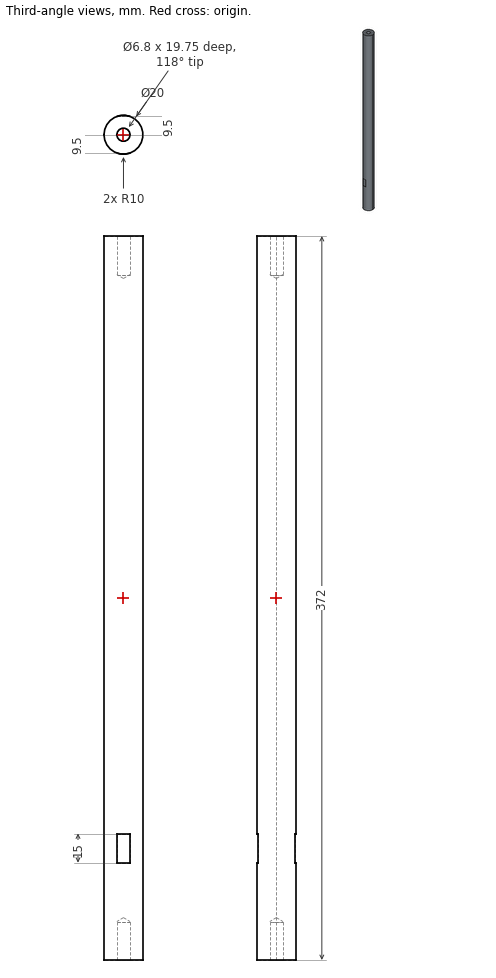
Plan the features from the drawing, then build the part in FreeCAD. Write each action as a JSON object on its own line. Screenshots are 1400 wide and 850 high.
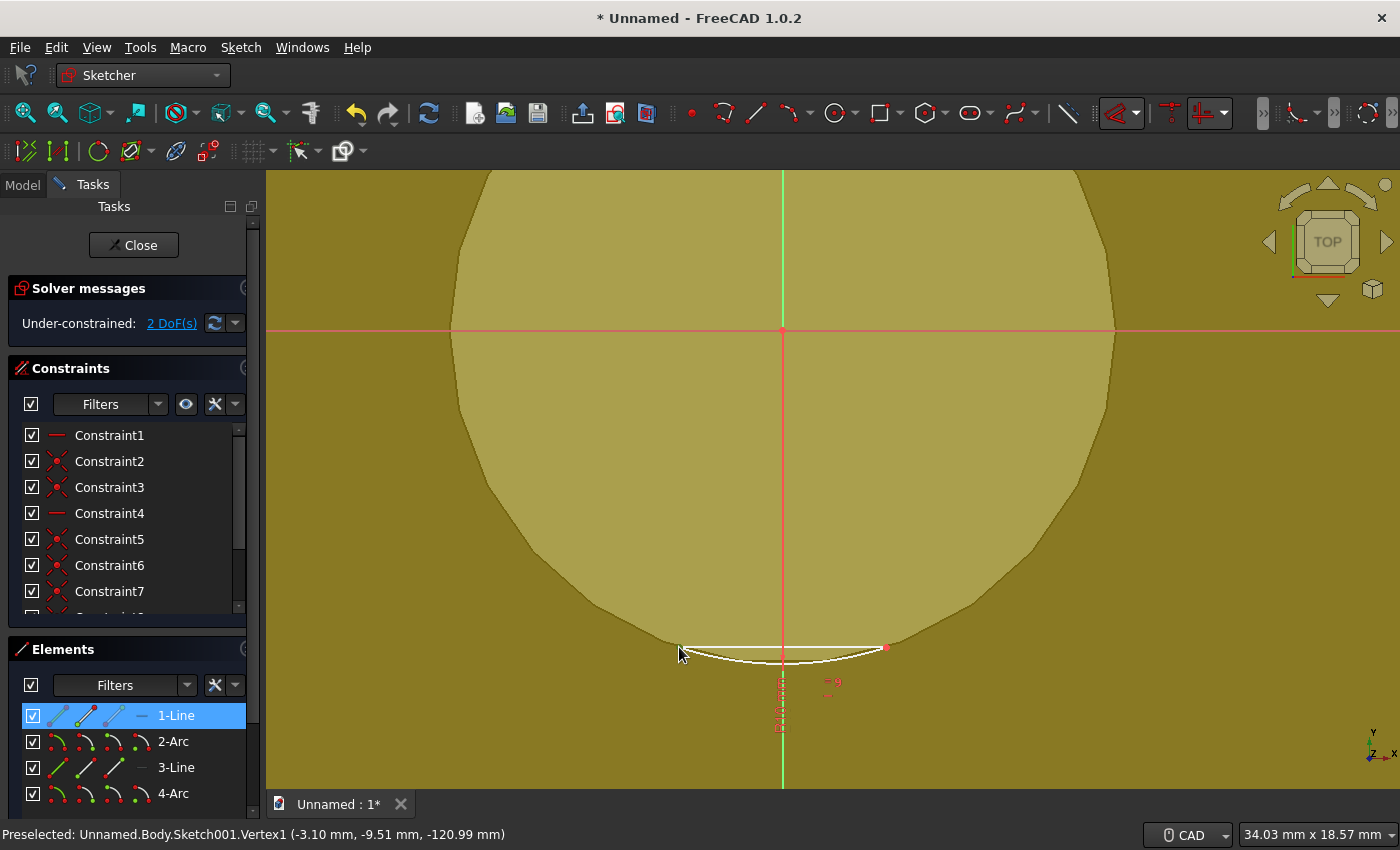
{"action": "key", "text": "i"}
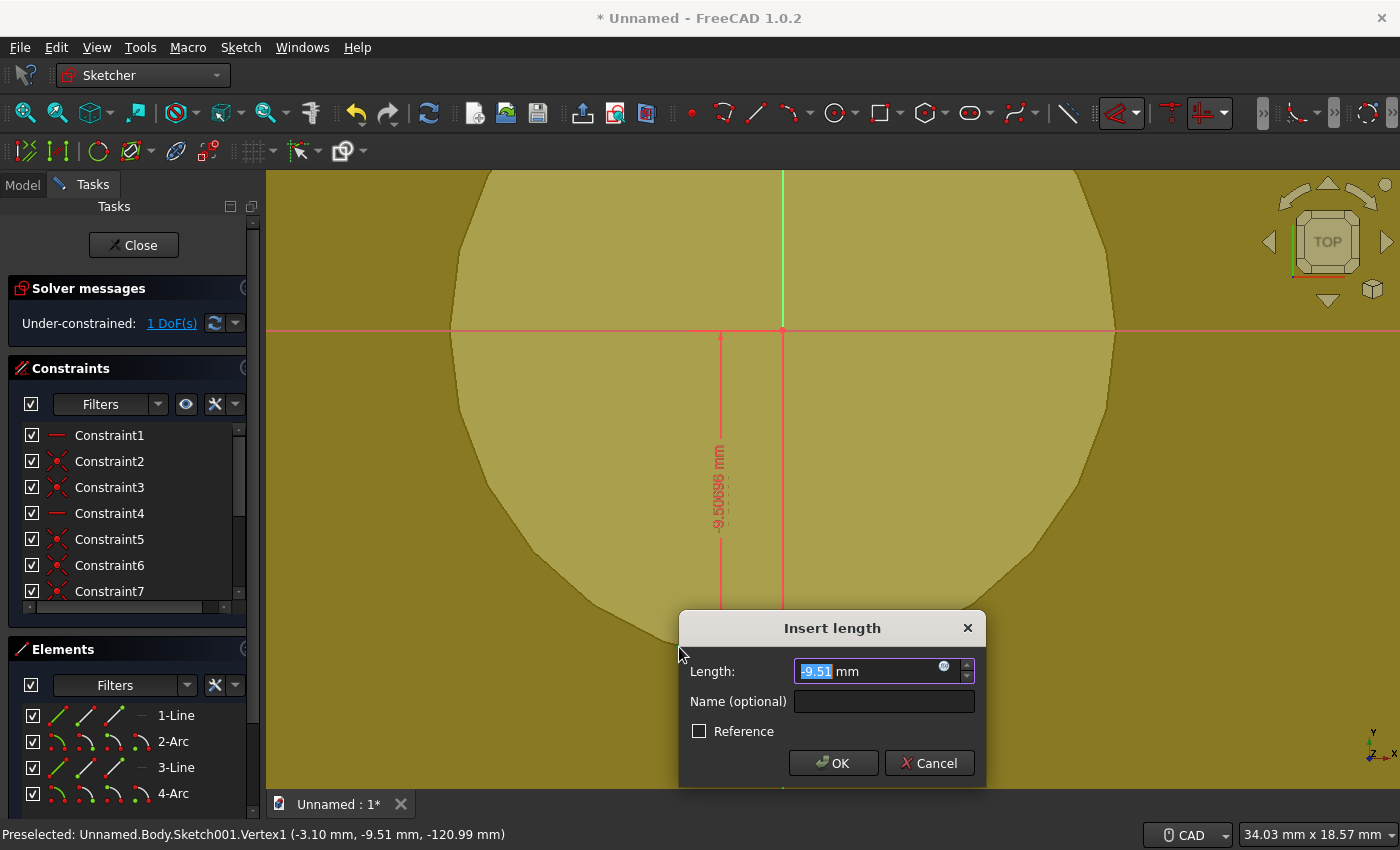
{"action": "type", "text": "-9.5"}
{"action": "key", "text": "Return"}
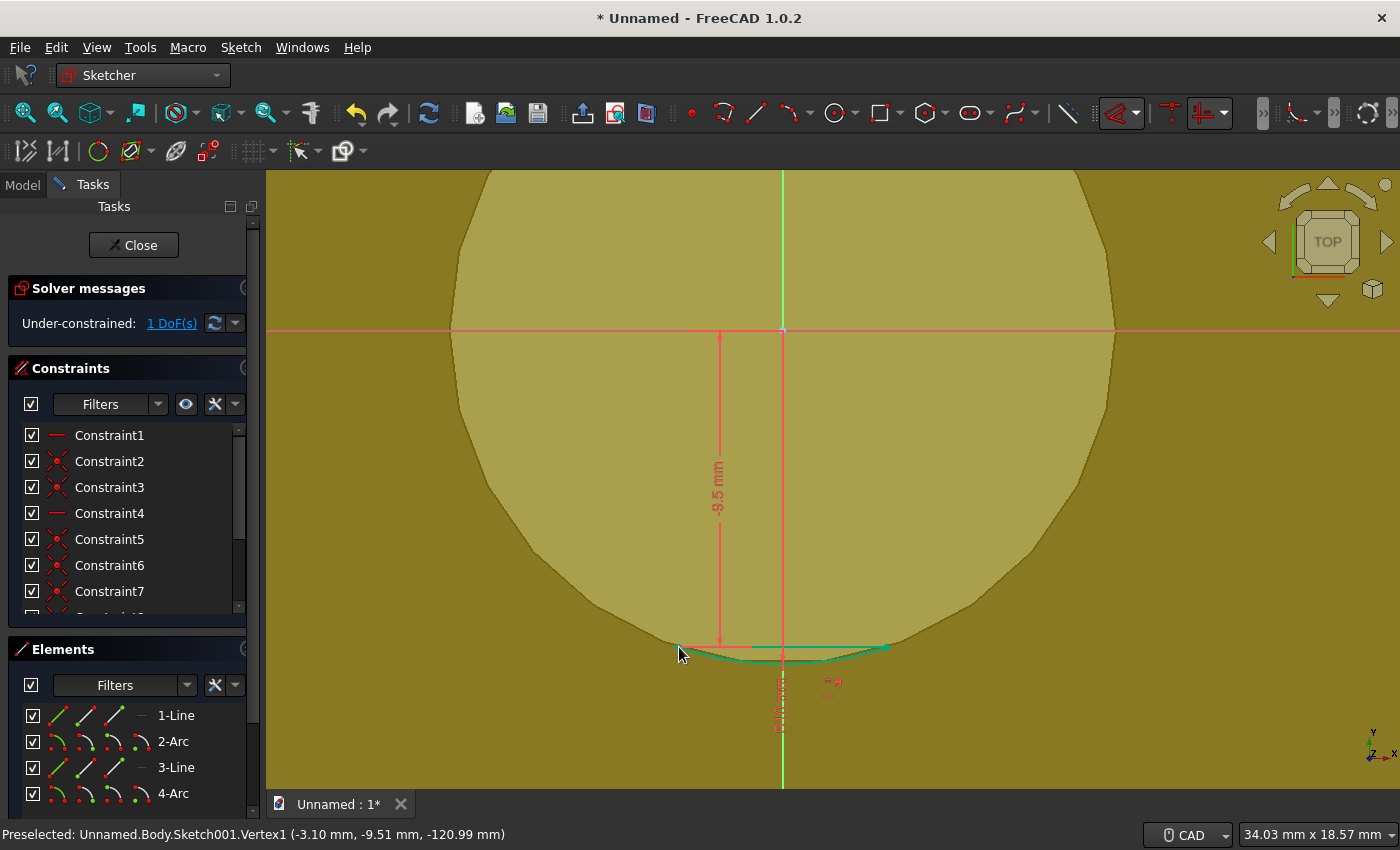
{"action": "scroll", "coordinate": [742, 661], "scroll_direction": "down", "scroll_amount": 3}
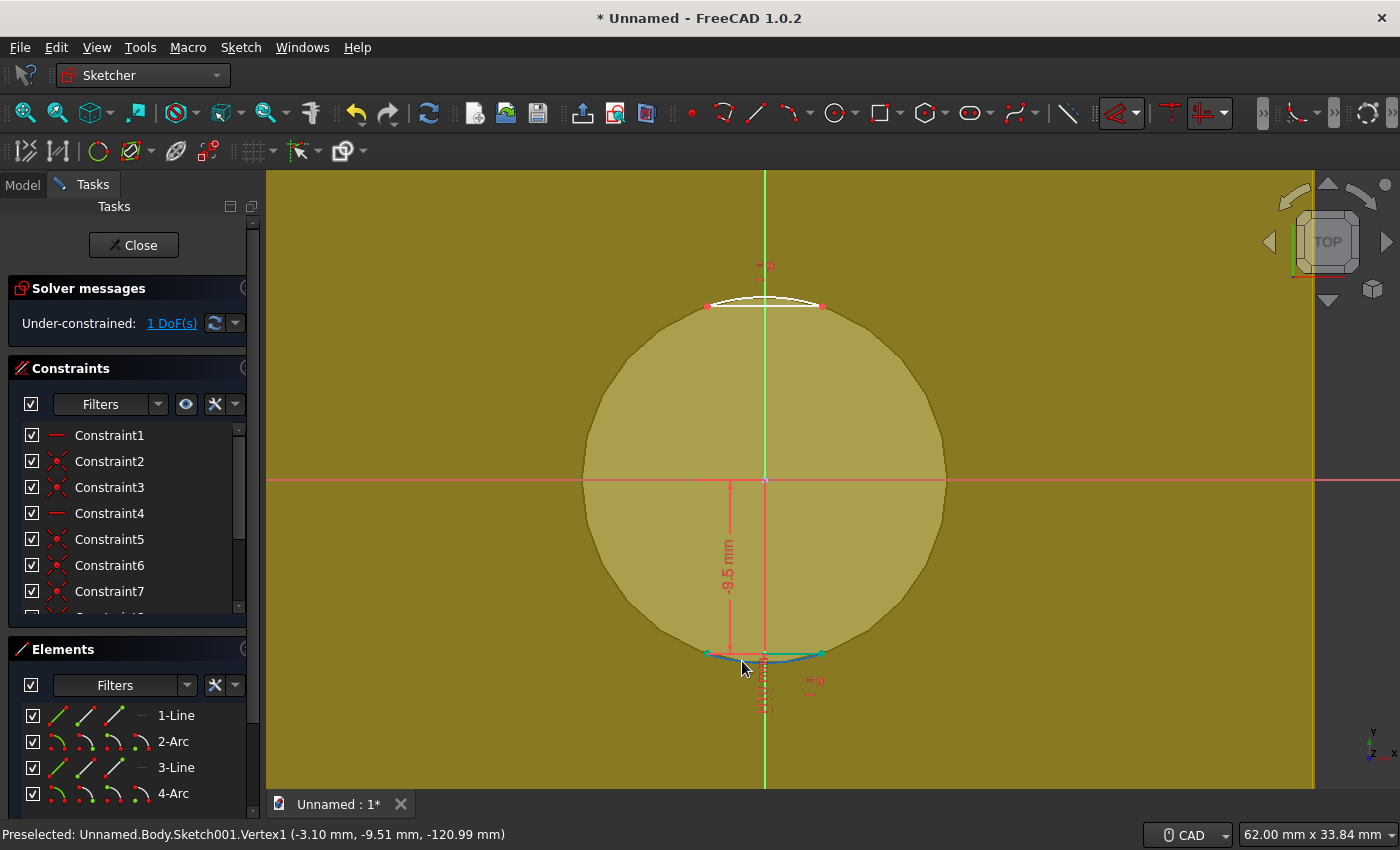
{"action": "left_click", "coordinate": [822, 306]}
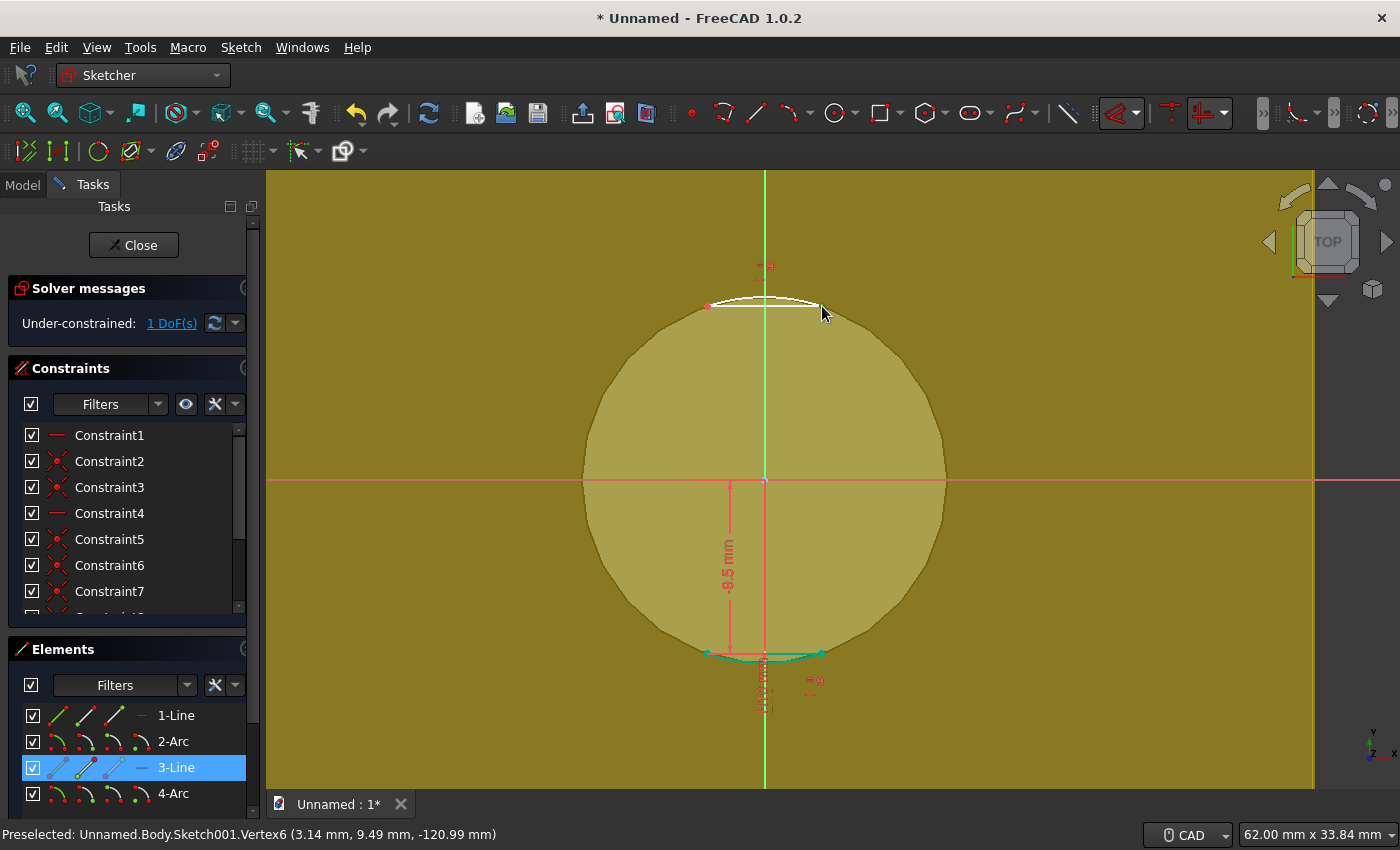
{"action": "left_click", "coordinate": [1138, 114]}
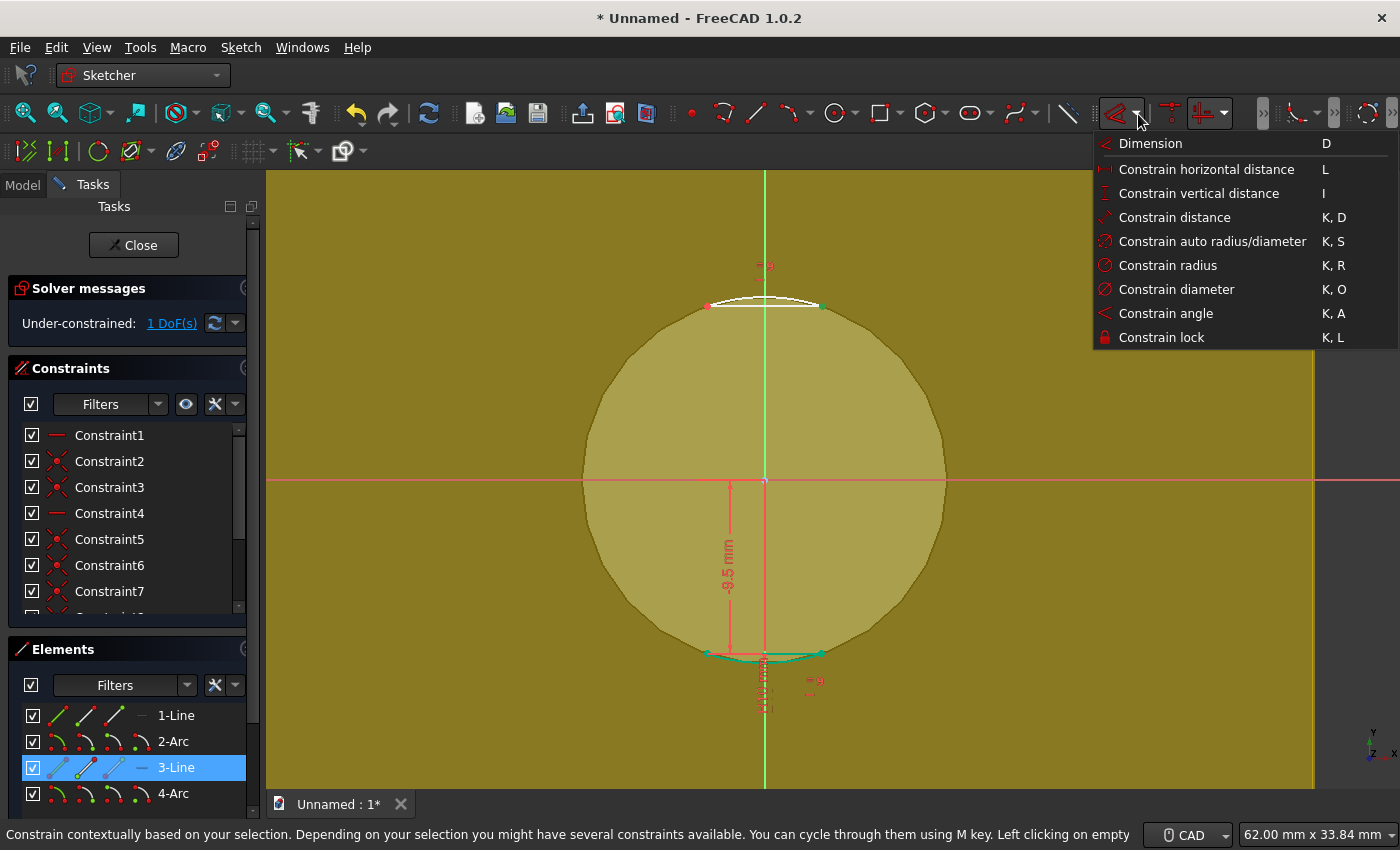
{"action": "left_click", "coordinate": [1246, 193]}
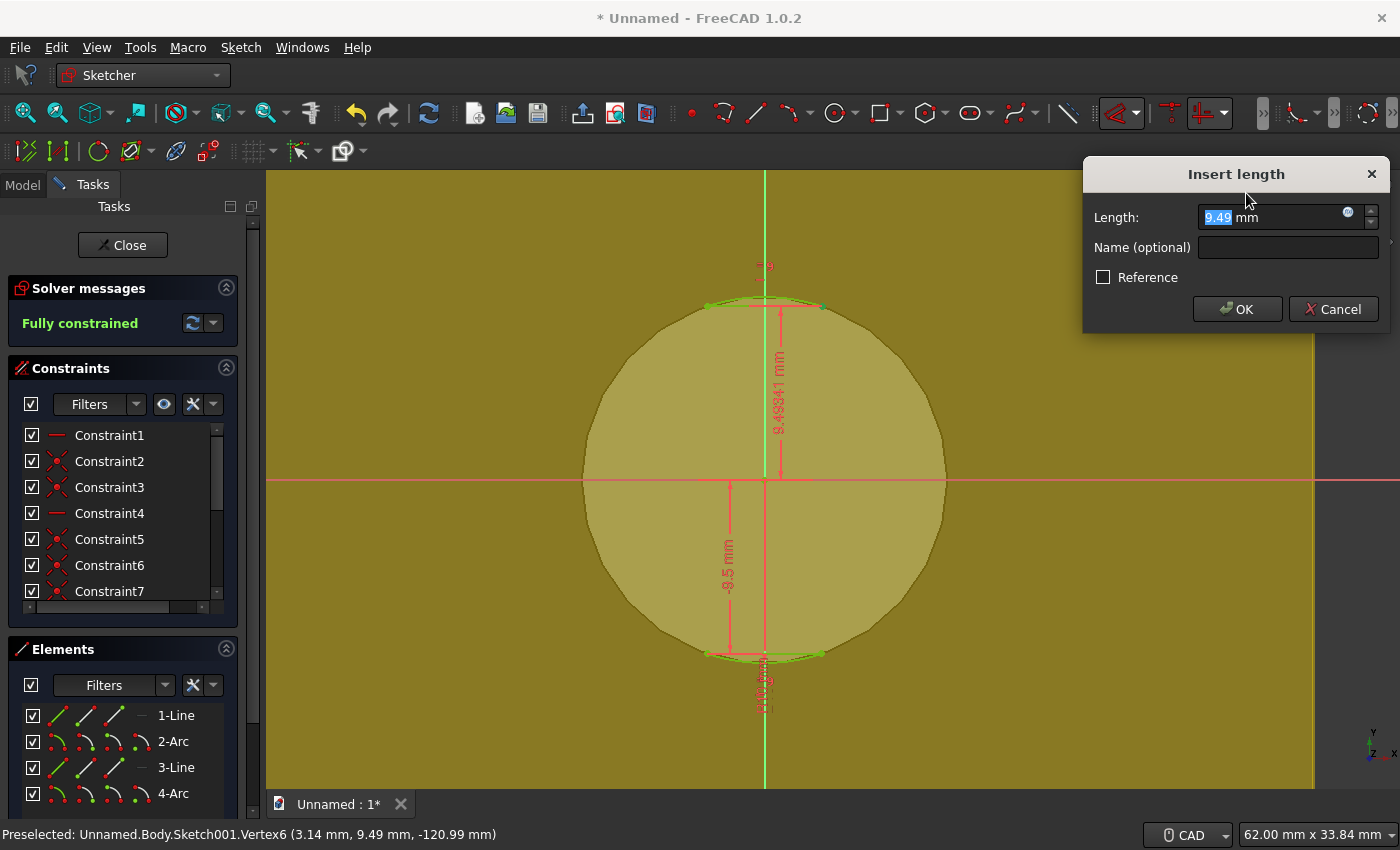
{"action": "type", "text": "9.5"}
{"action": "key", "text": "Return"}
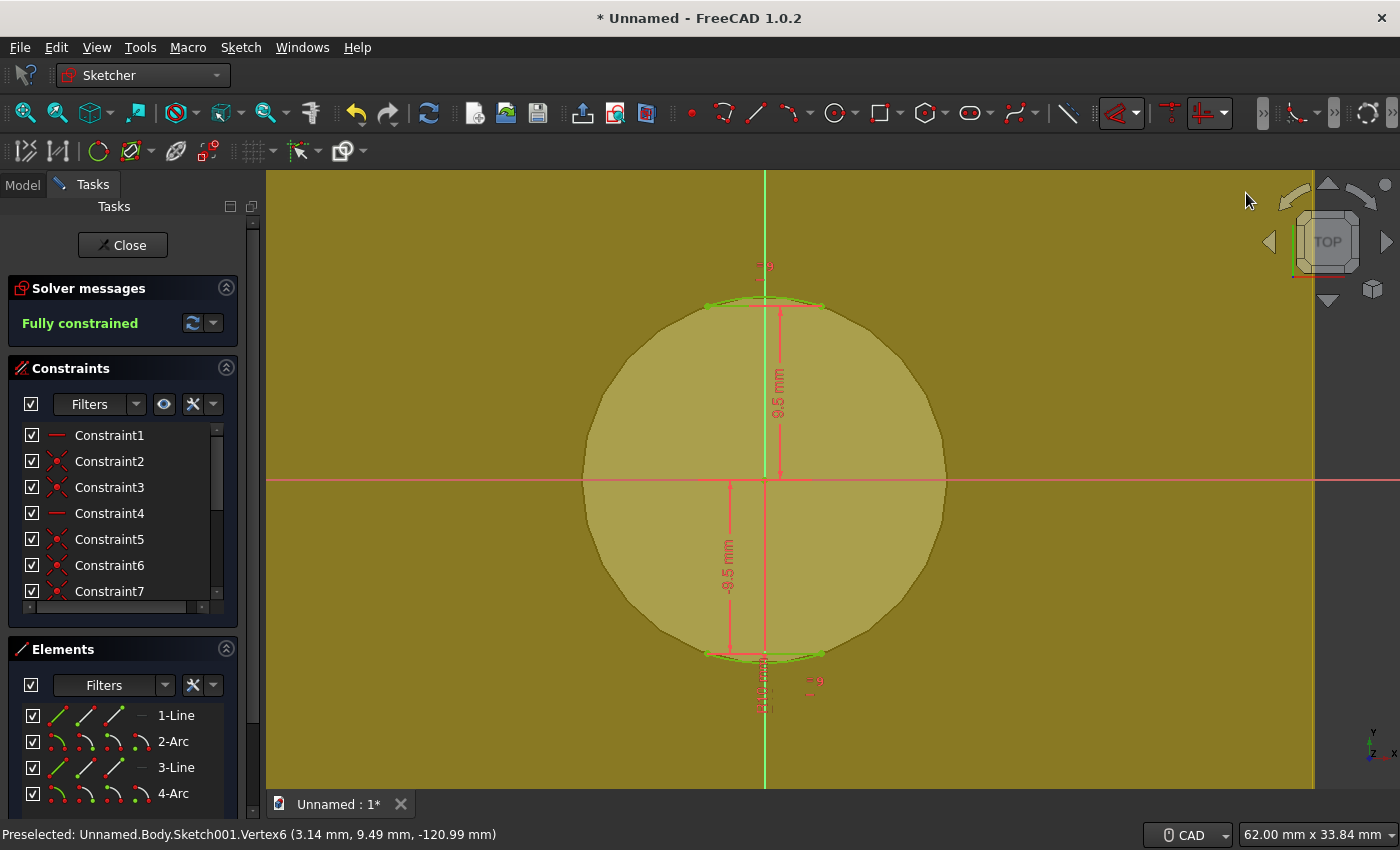
{"action": "left_click", "coordinate": [123, 245]}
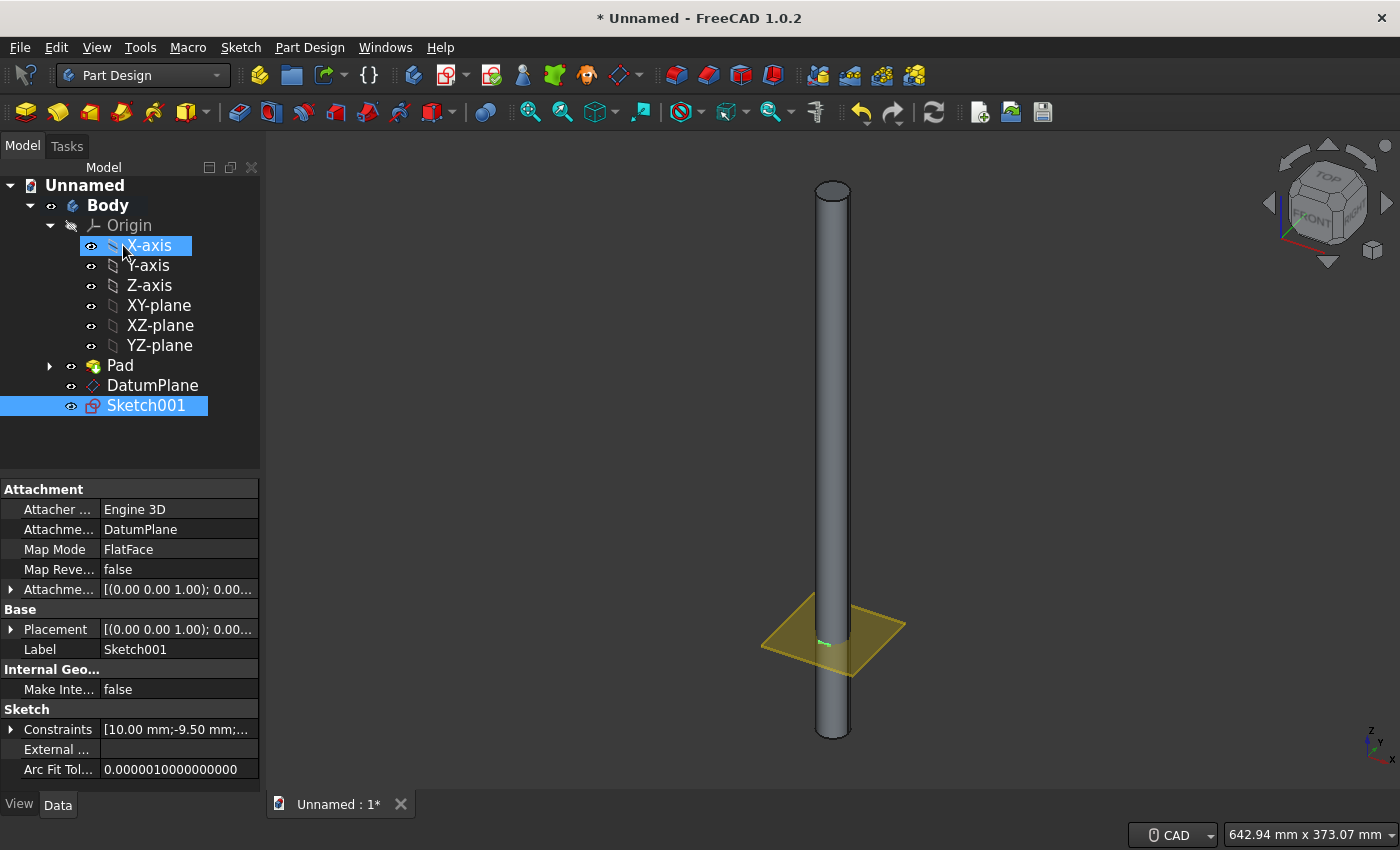
{"action": "left_click", "coordinate": [240, 112]}